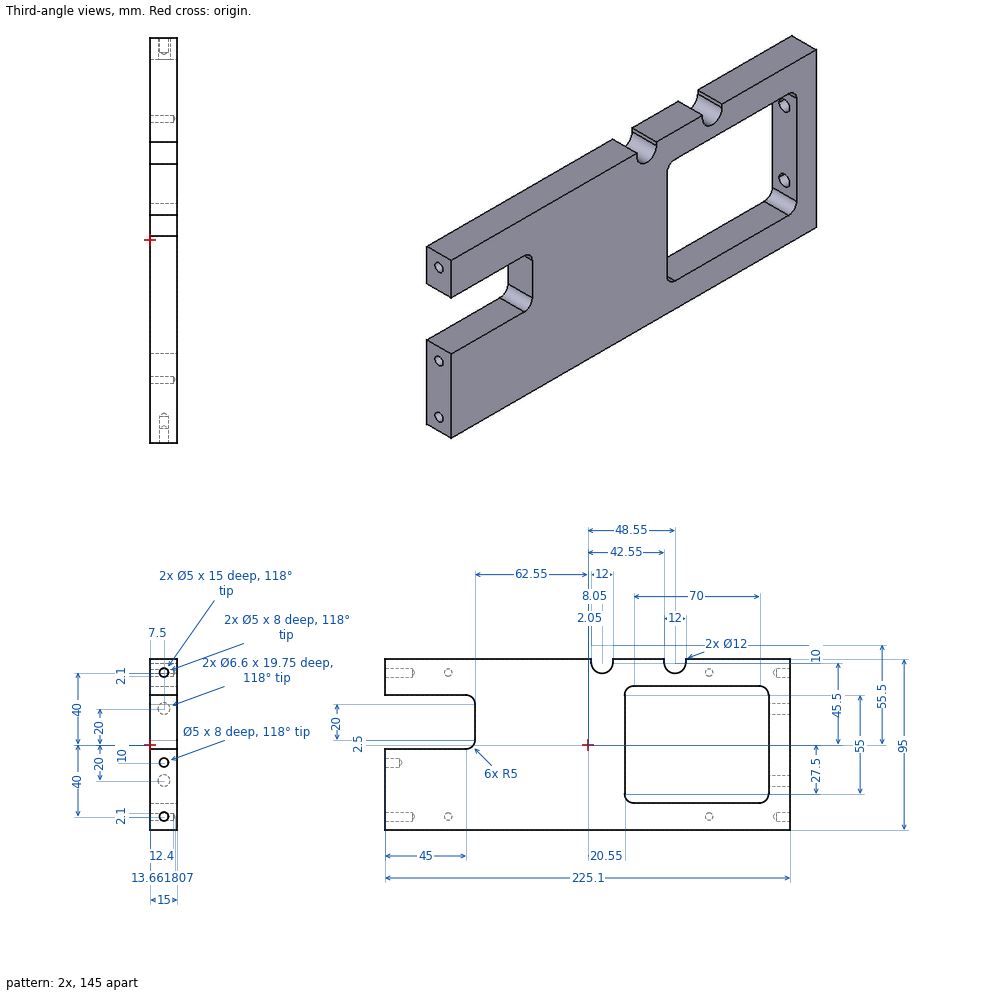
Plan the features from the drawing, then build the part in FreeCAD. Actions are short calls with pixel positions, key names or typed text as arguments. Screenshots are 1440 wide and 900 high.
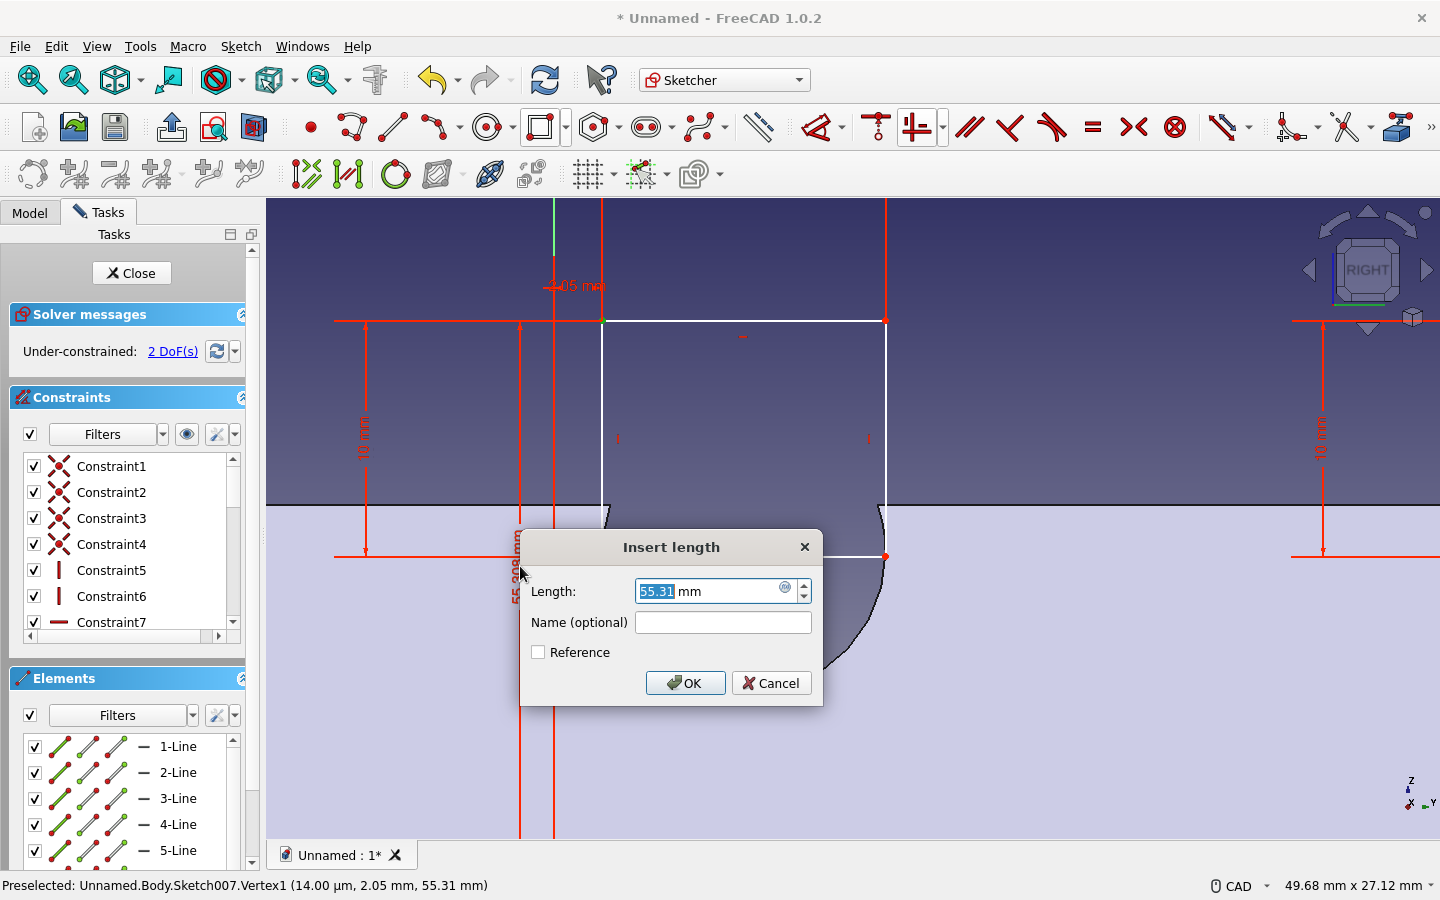
text(55.5)
key(Return)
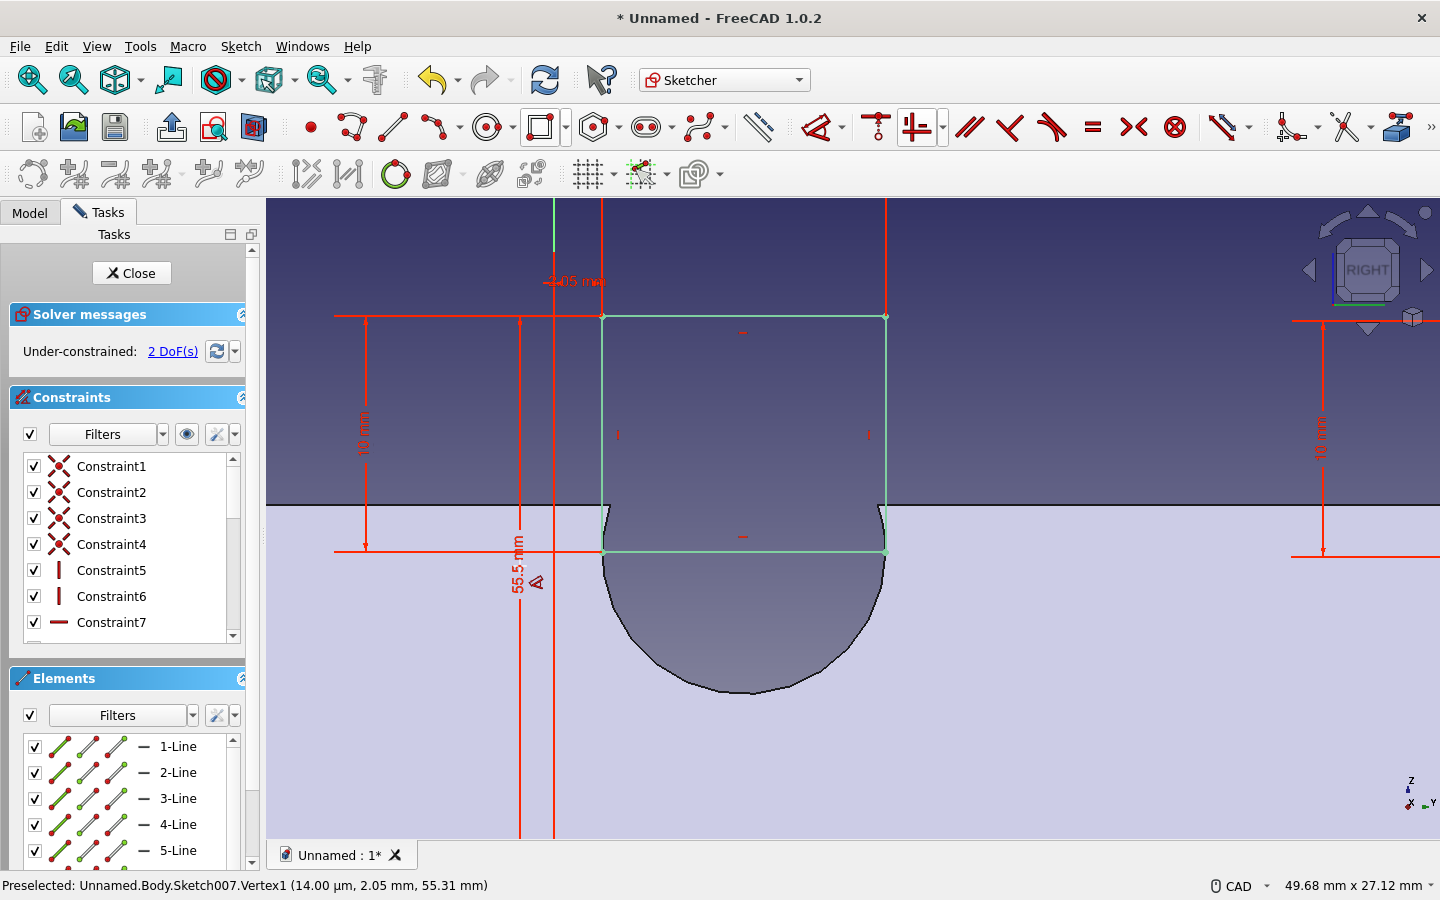
scroll(606, 323, down, 6)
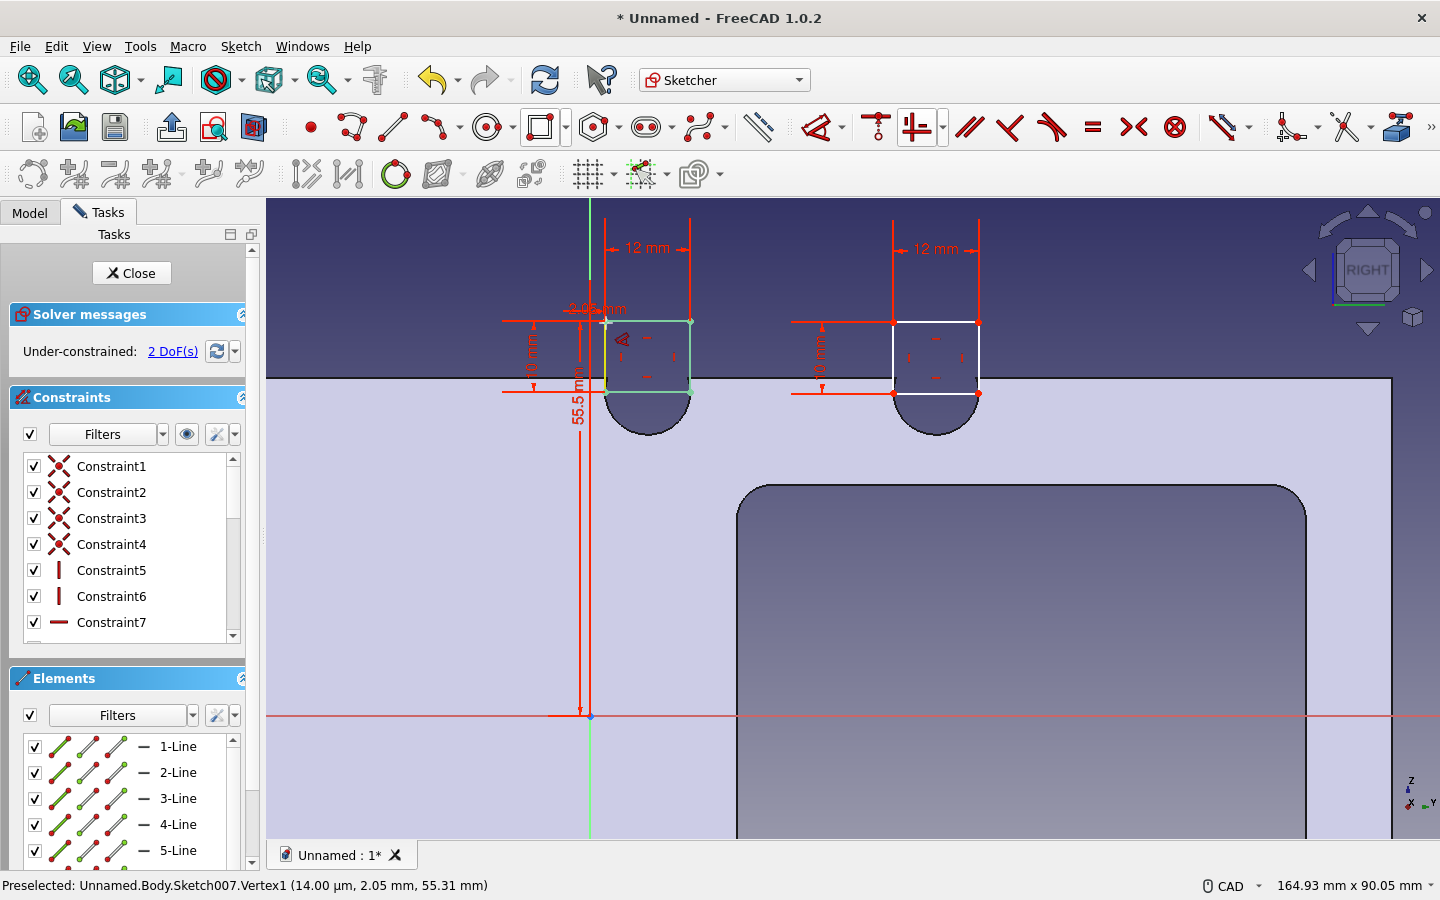
click(893, 322)
click(556, 519)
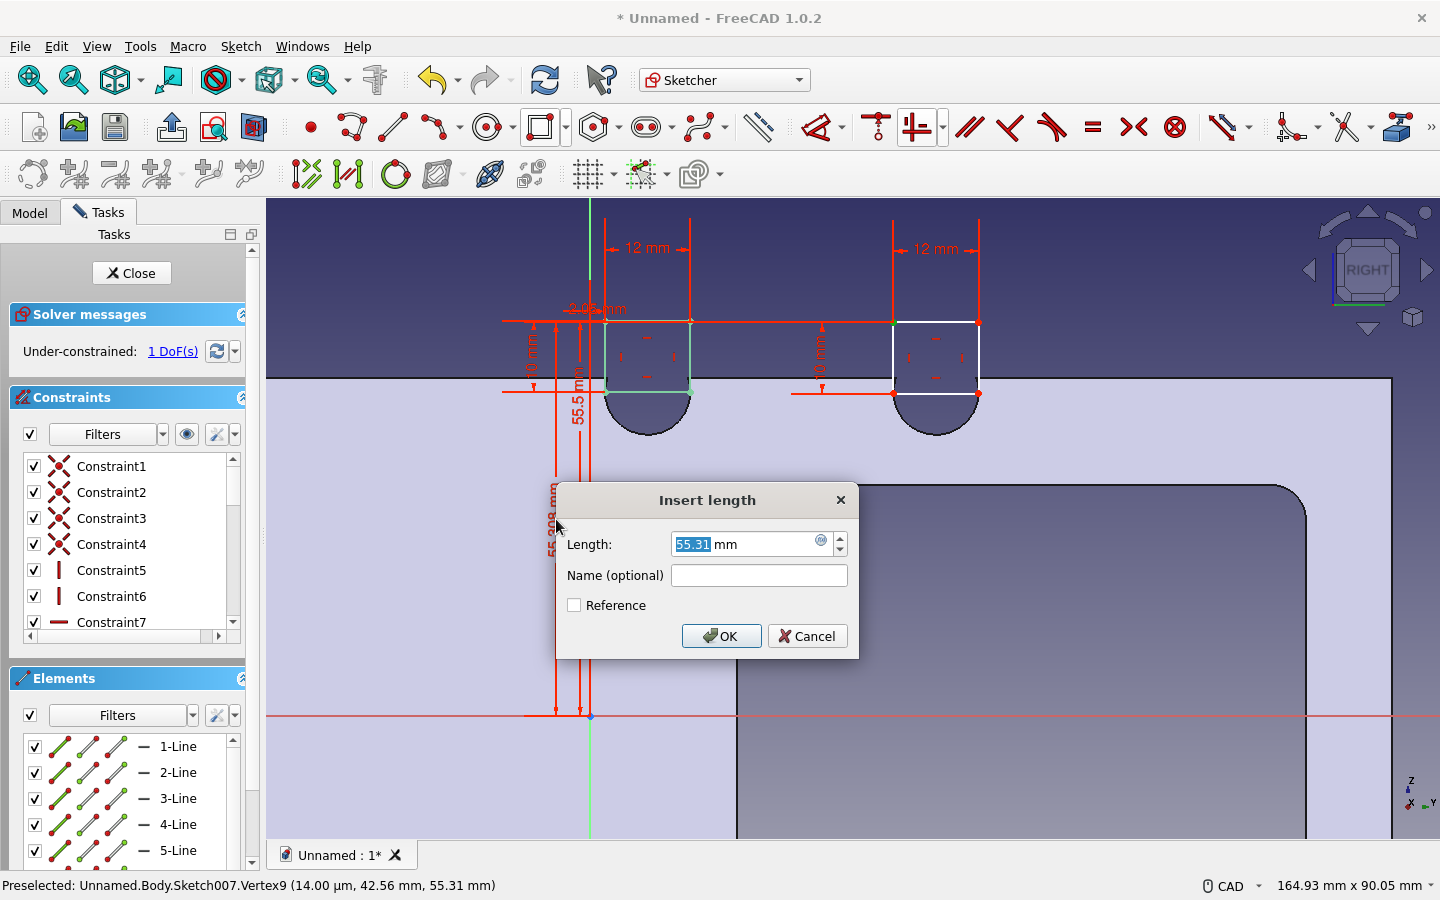
text(55.5)
key(Return)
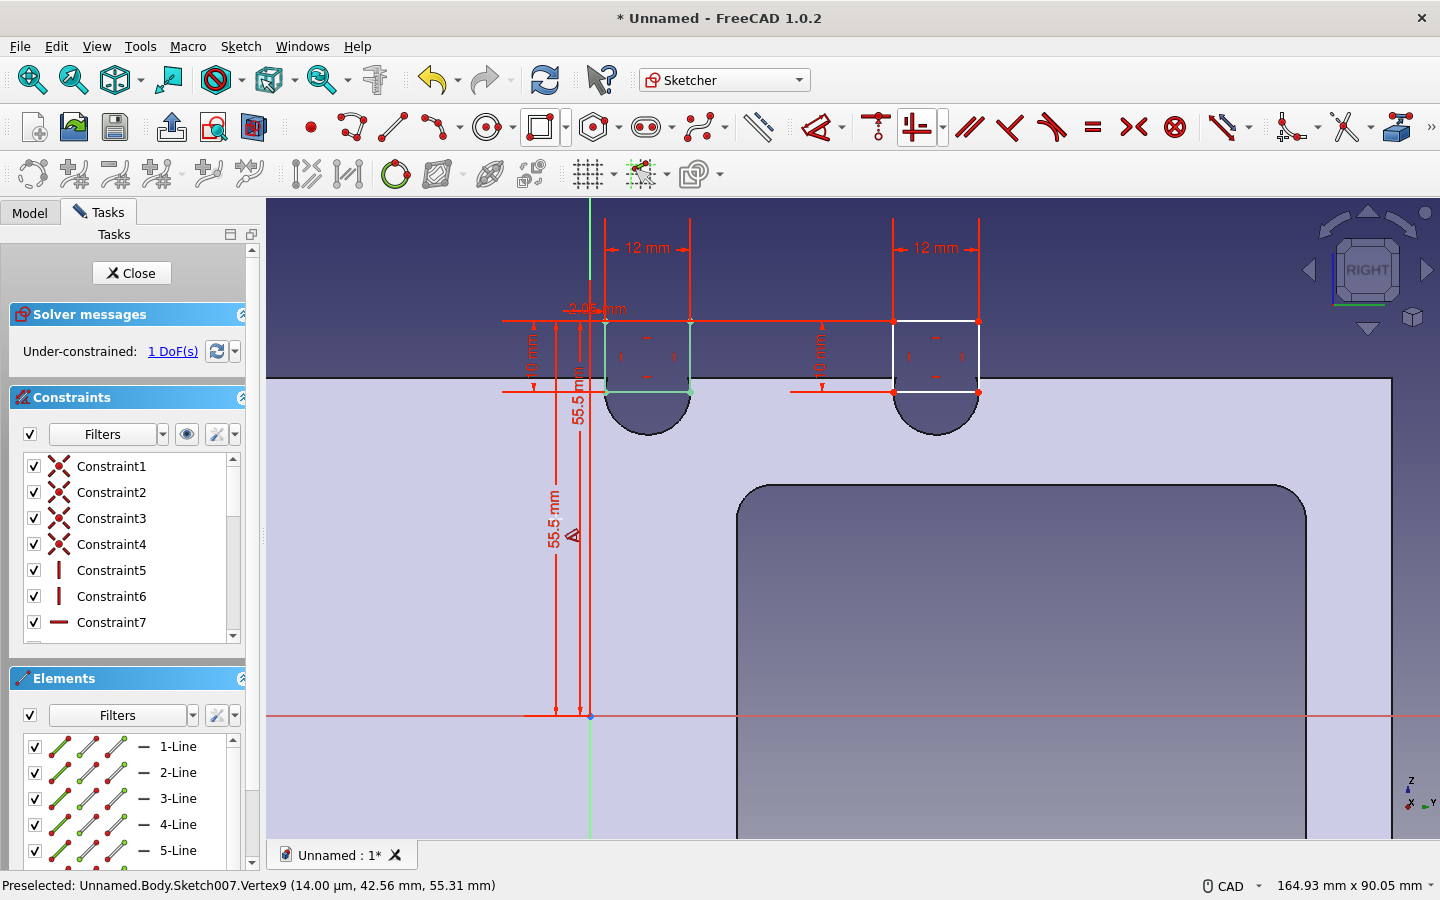
click(893, 321)
click(742, 750)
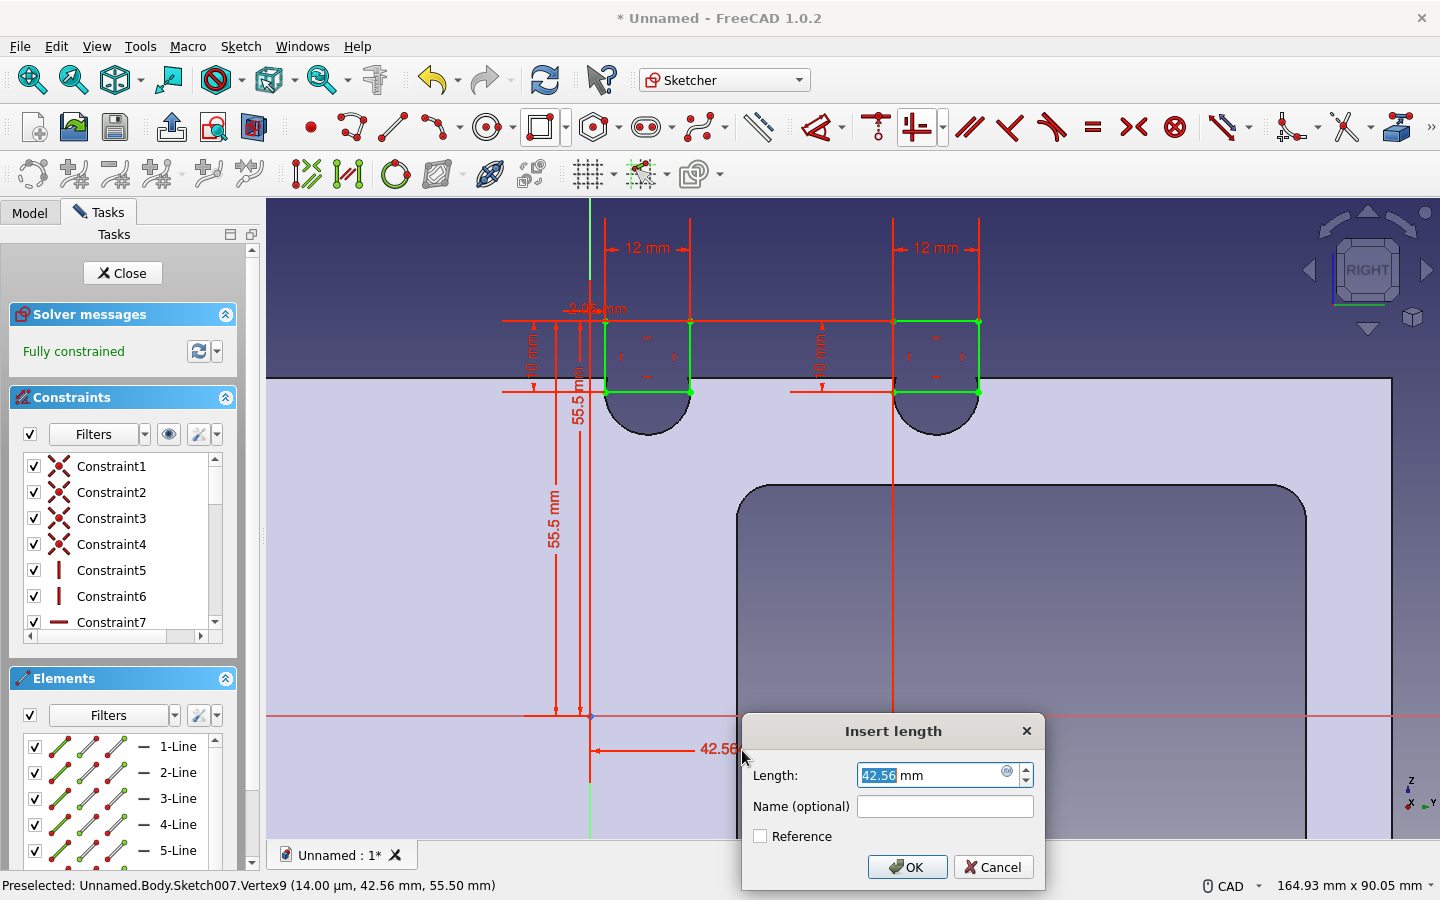
text(42.55)
key(Return)
key(Escape)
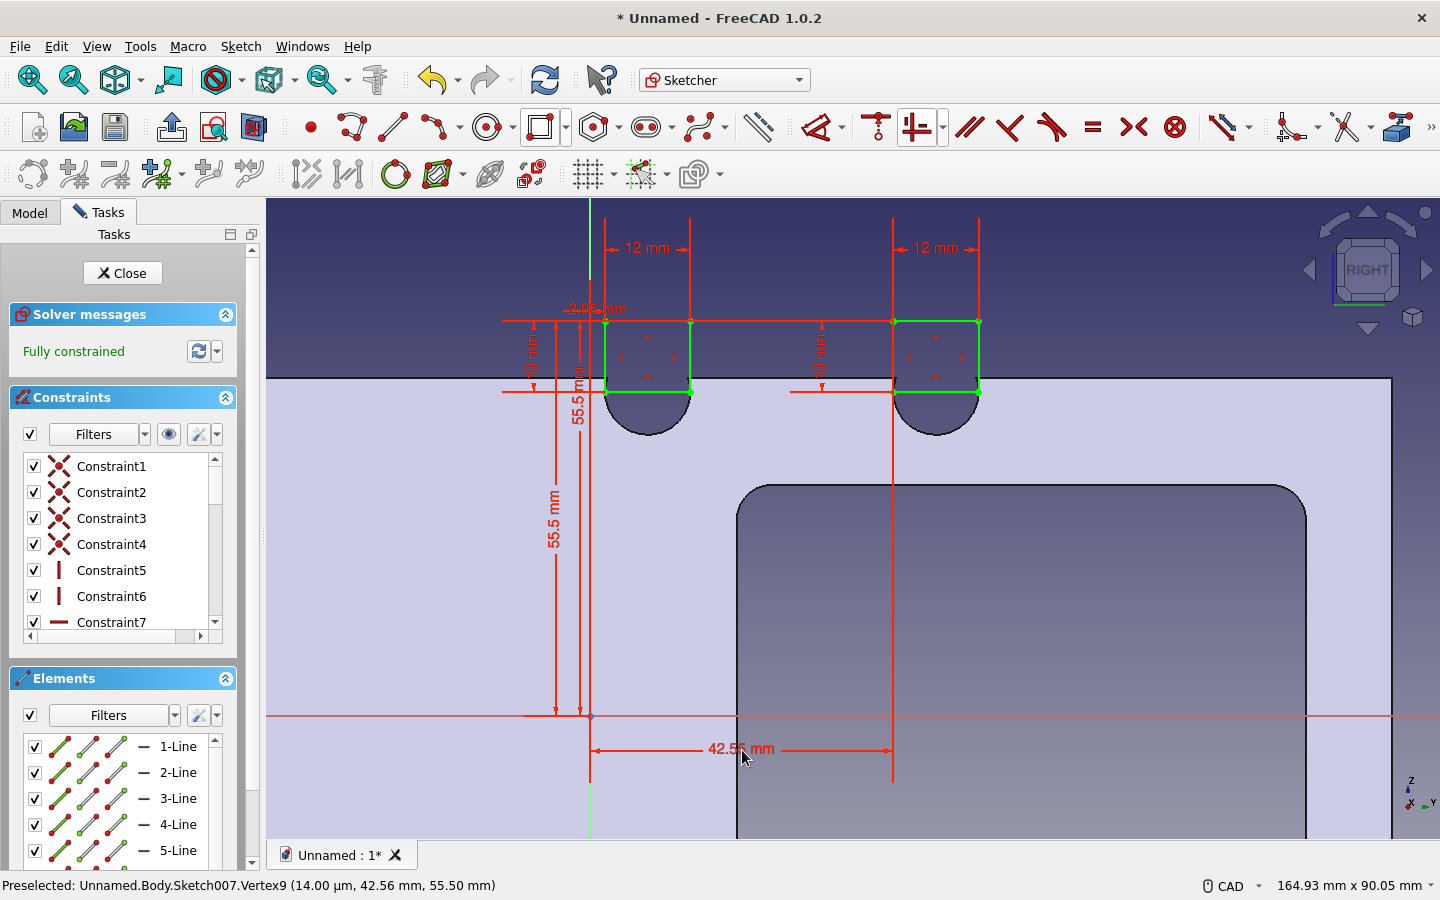
click(123, 273)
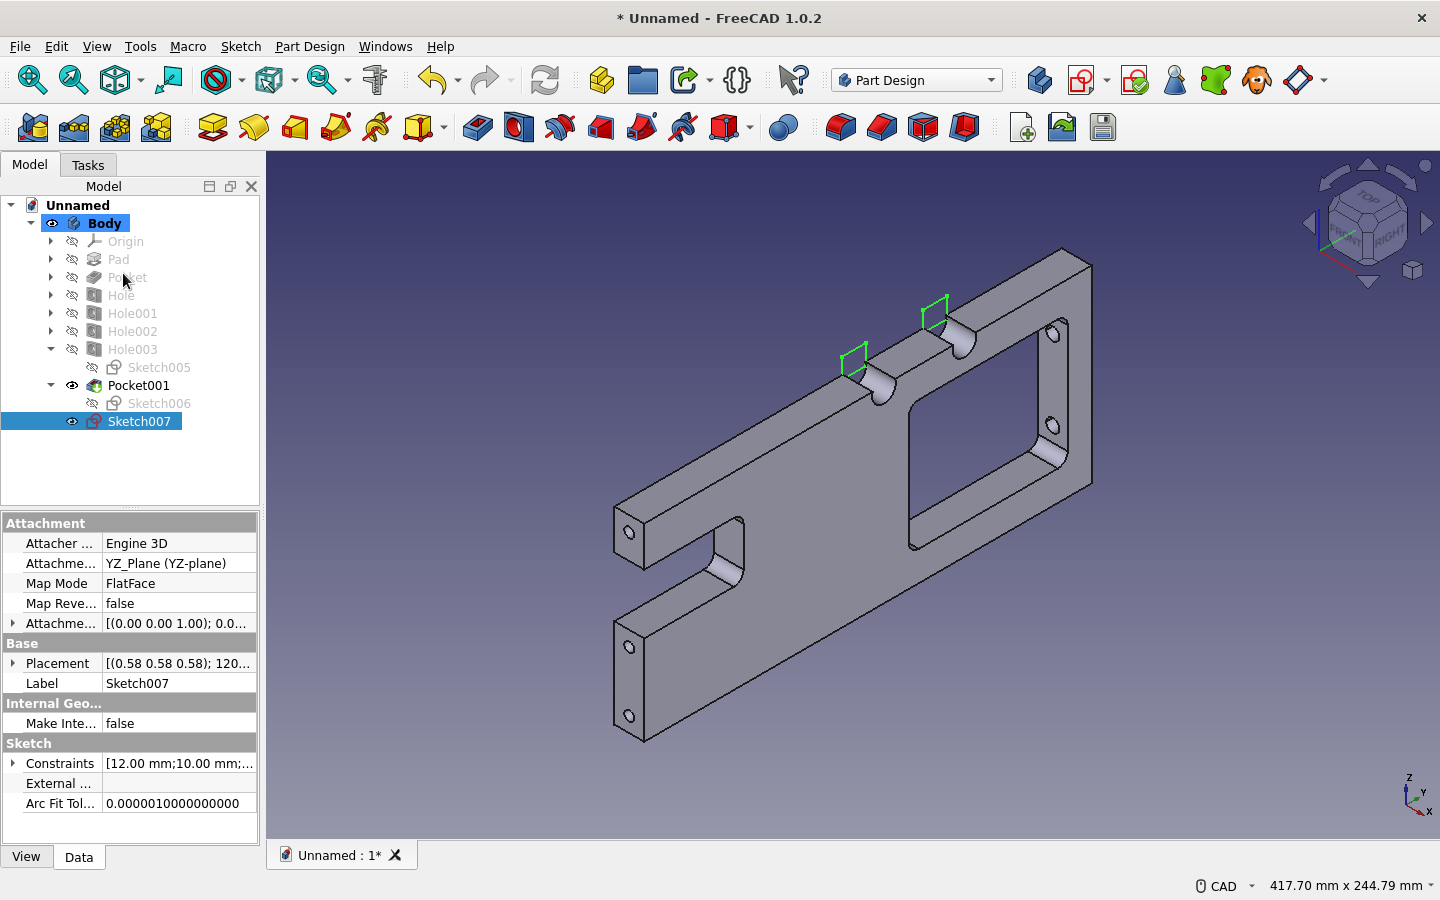
click(478, 128)